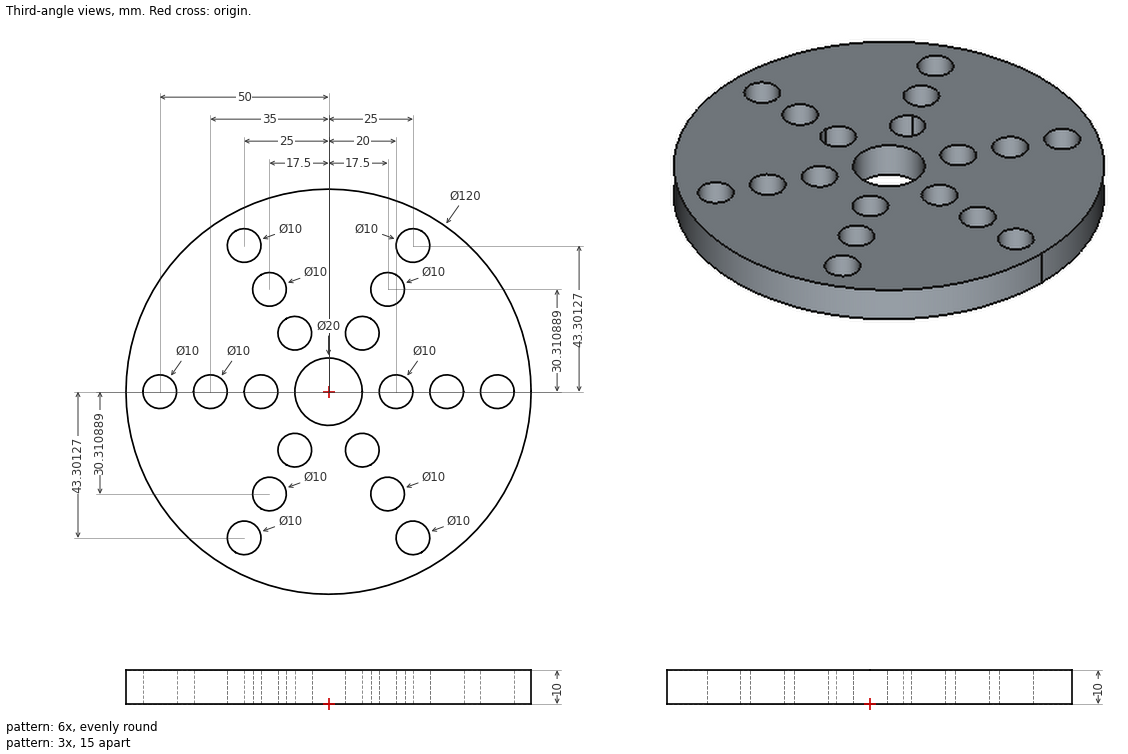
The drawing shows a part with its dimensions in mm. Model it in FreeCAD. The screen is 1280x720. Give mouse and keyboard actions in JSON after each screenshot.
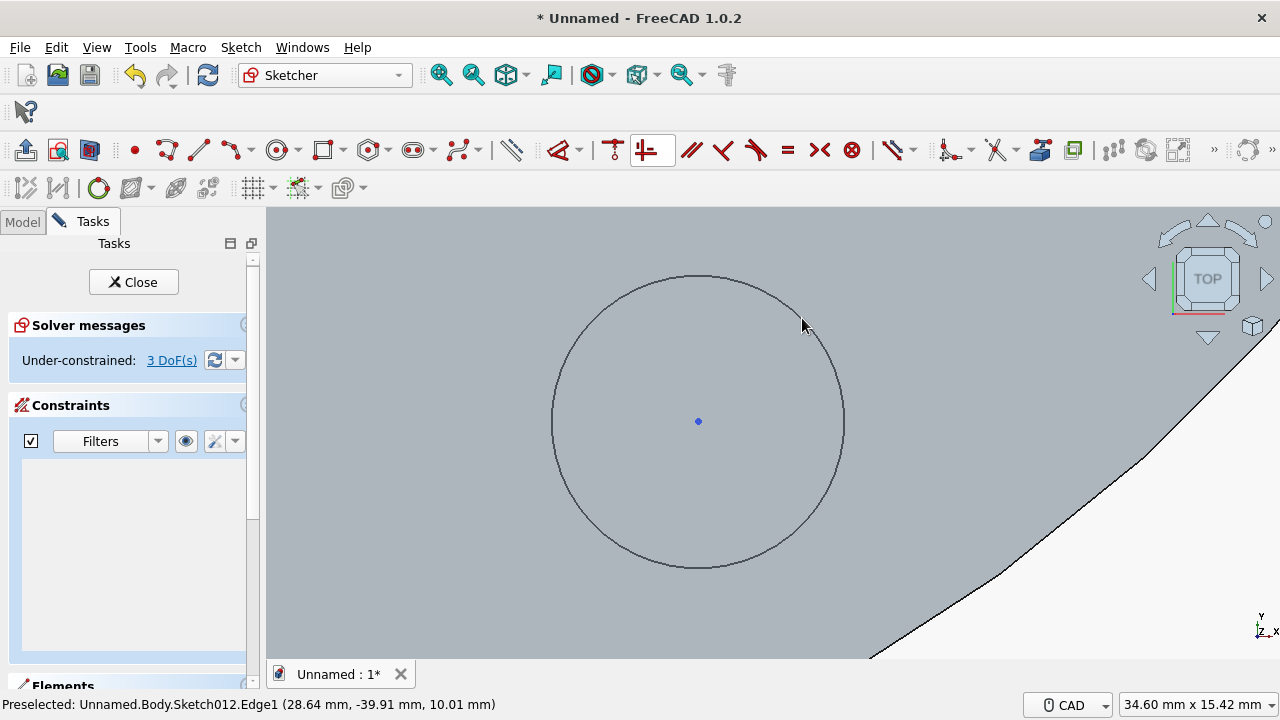
{"action": "left_click", "coordinate": [558, 150]}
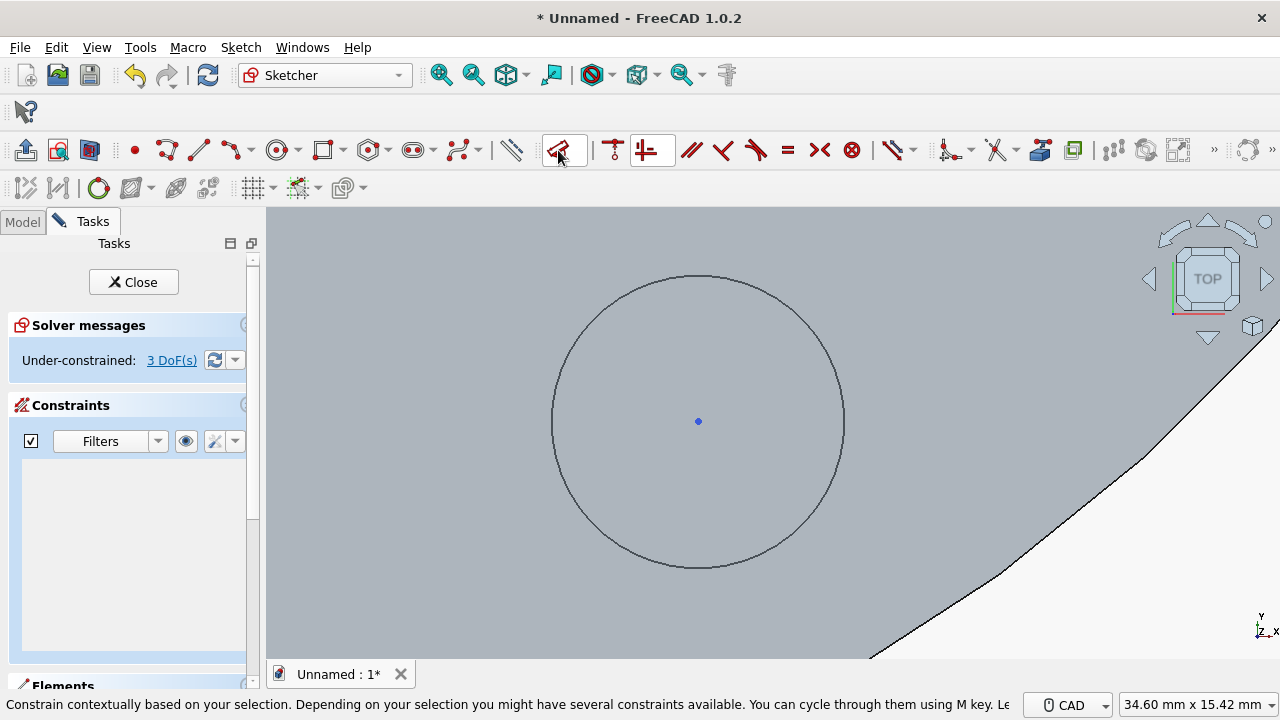
{"action": "left_click", "coordinate": [801, 318]}
{"action": "left_click", "coordinate": [824, 295]}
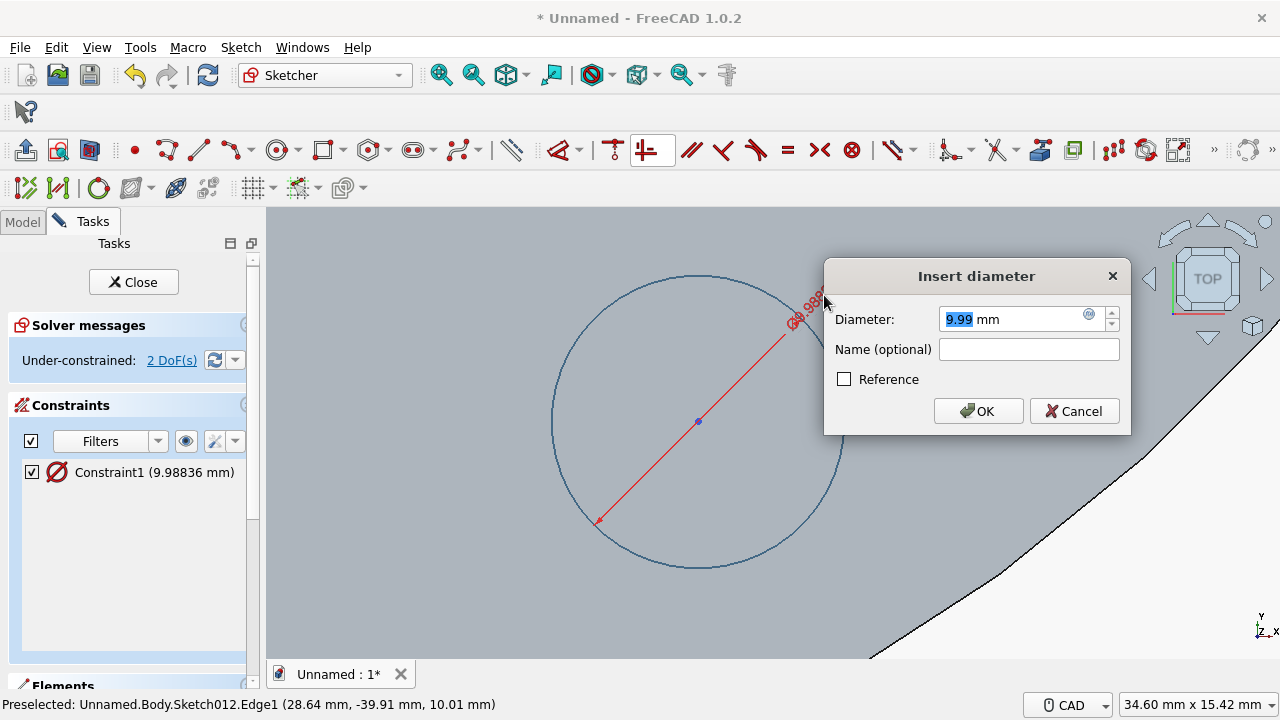
{"action": "type", "text": "10"}
{"action": "key", "text": "Return"}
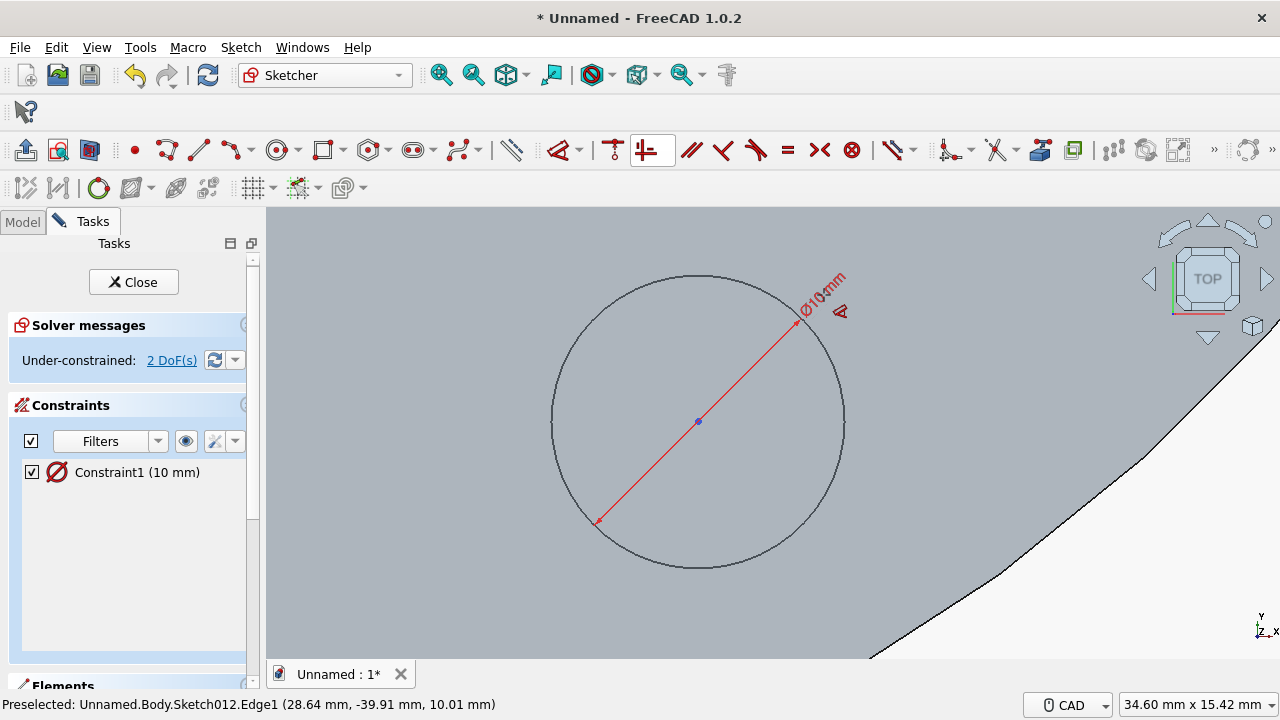
{"action": "left_click", "coordinate": [698, 422]}
{"action": "left_click", "coordinate": [496, 456]}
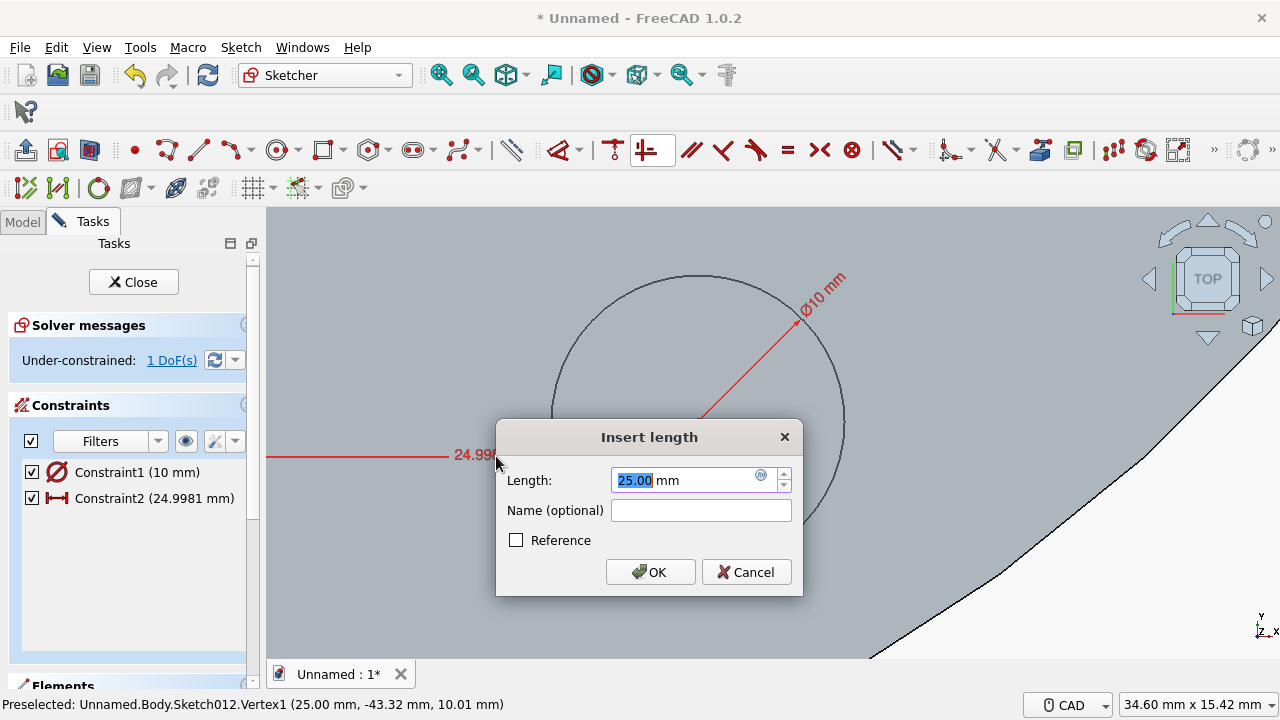
{"action": "type", "text": "25"}
{"action": "key", "text": "Return"}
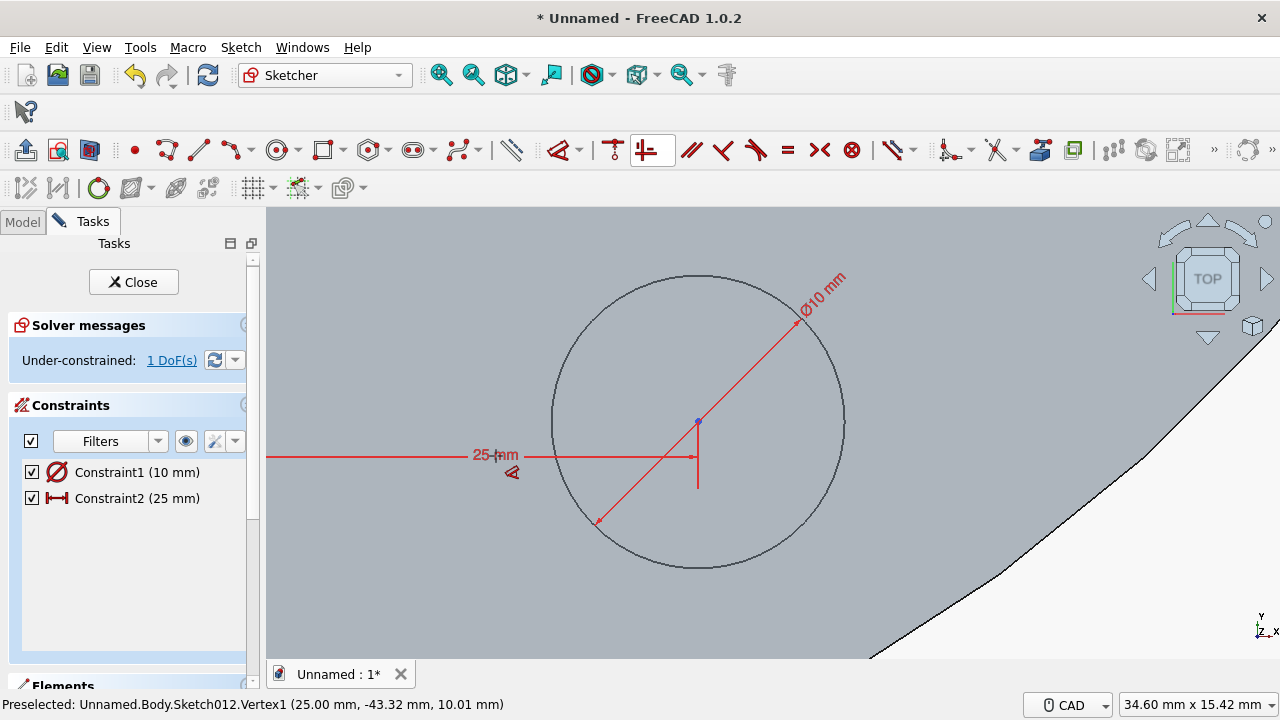
{"action": "left_click", "coordinate": [698, 422]}
{"action": "left_click", "coordinate": [732, 328]}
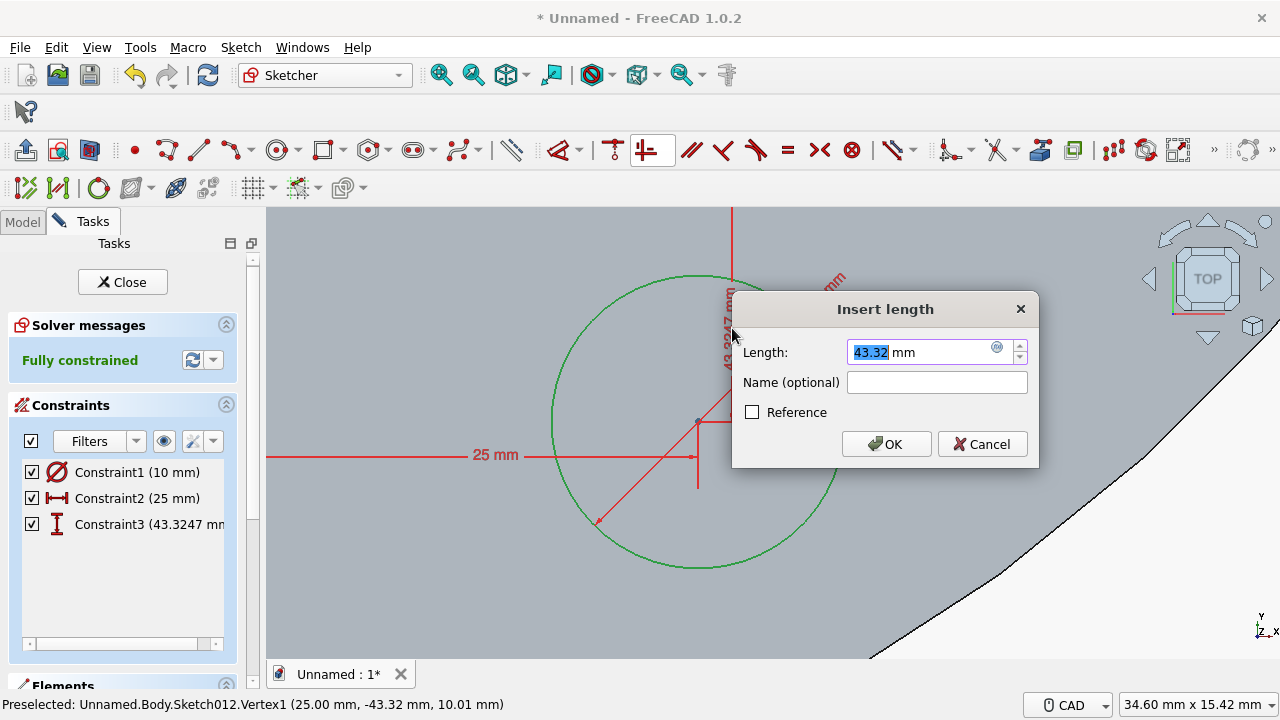
{"action": "type", "text": "43.30127"}
{"action": "key", "text": "Return"}
{"action": "key", "text": "Escape"}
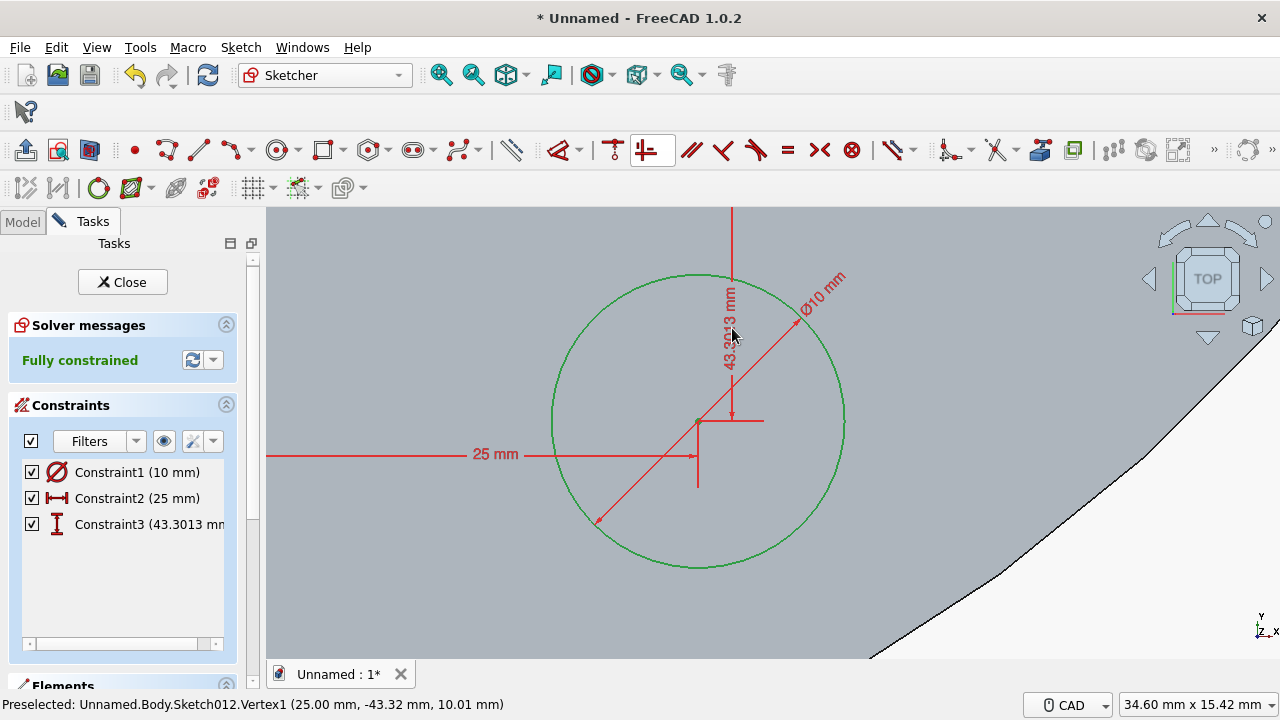
{"action": "left_click", "coordinate": [123, 282]}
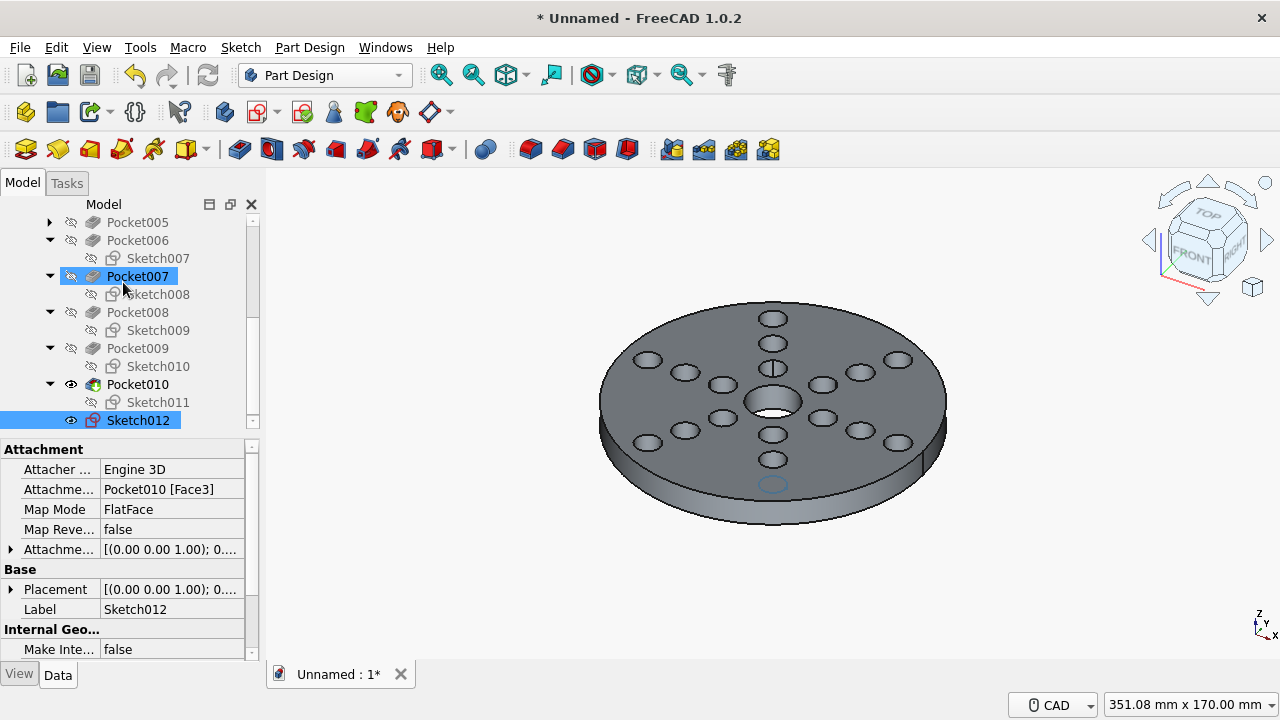
{"action": "left_click", "coordinate": [240, 150]}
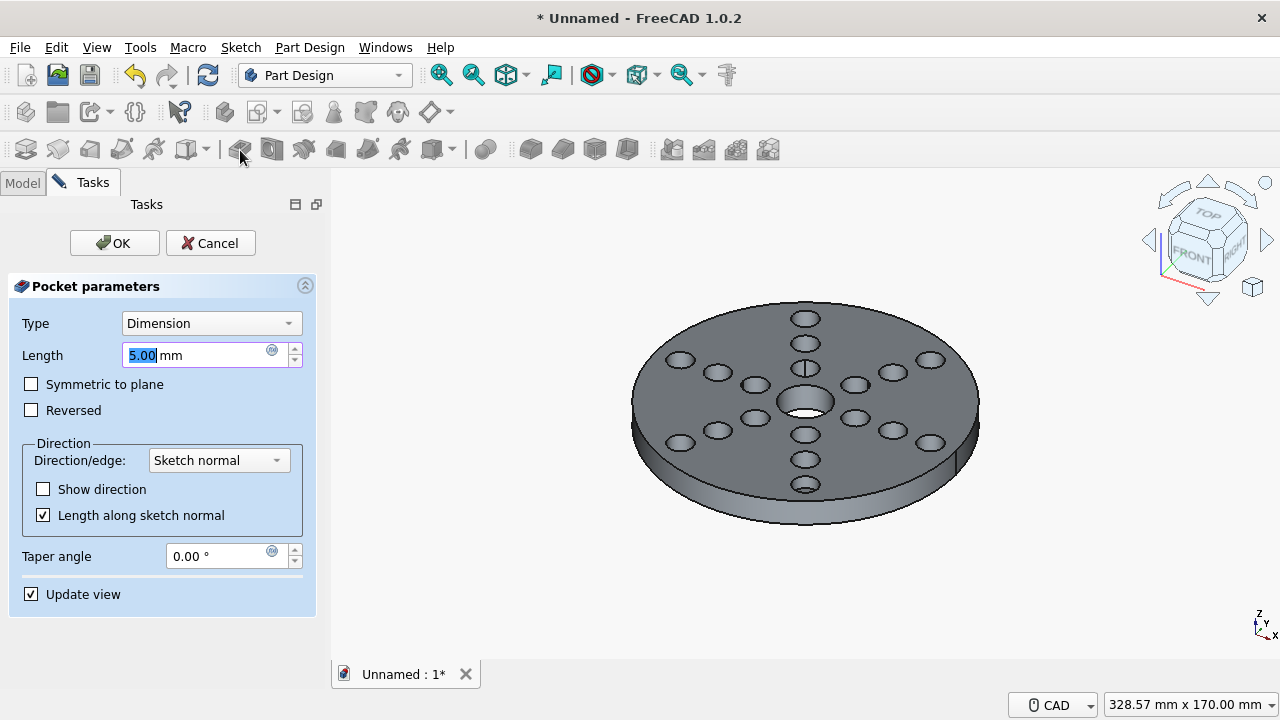
{"action": "type", "text": "10"}
{"action": "key", "text": "Tab"}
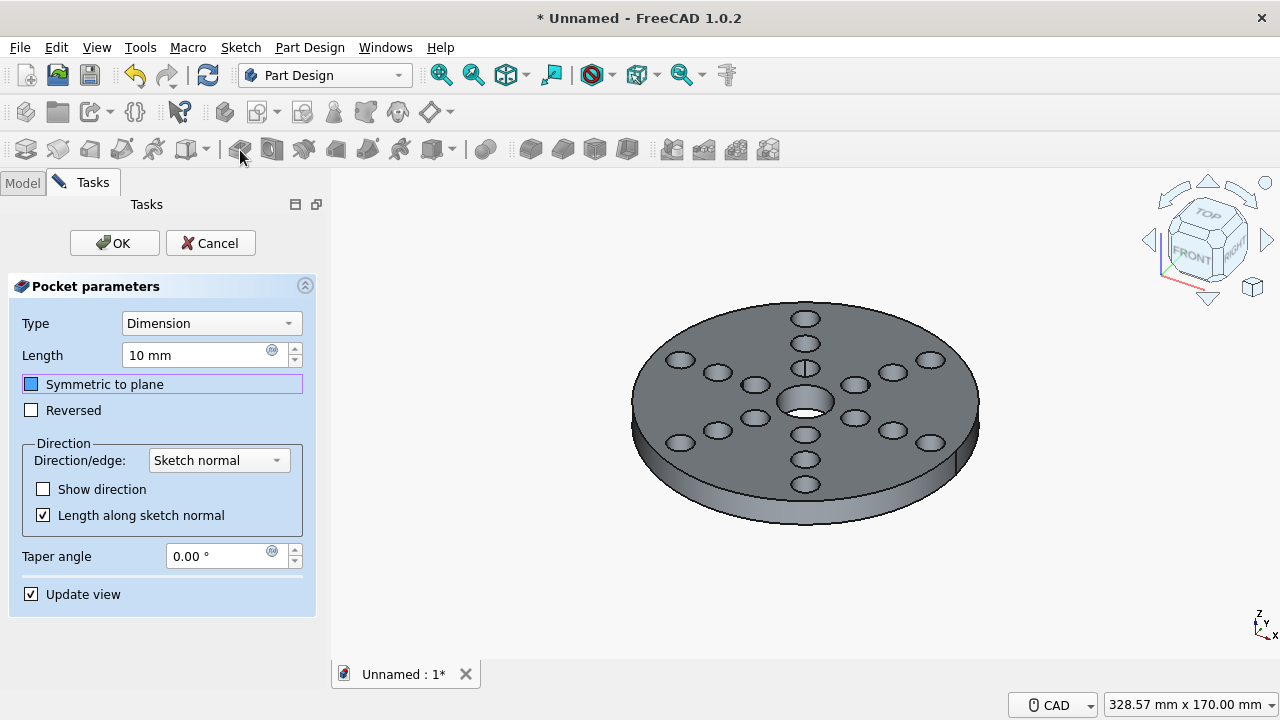
{"action": "left_click", "coordinate": [115, 243]}